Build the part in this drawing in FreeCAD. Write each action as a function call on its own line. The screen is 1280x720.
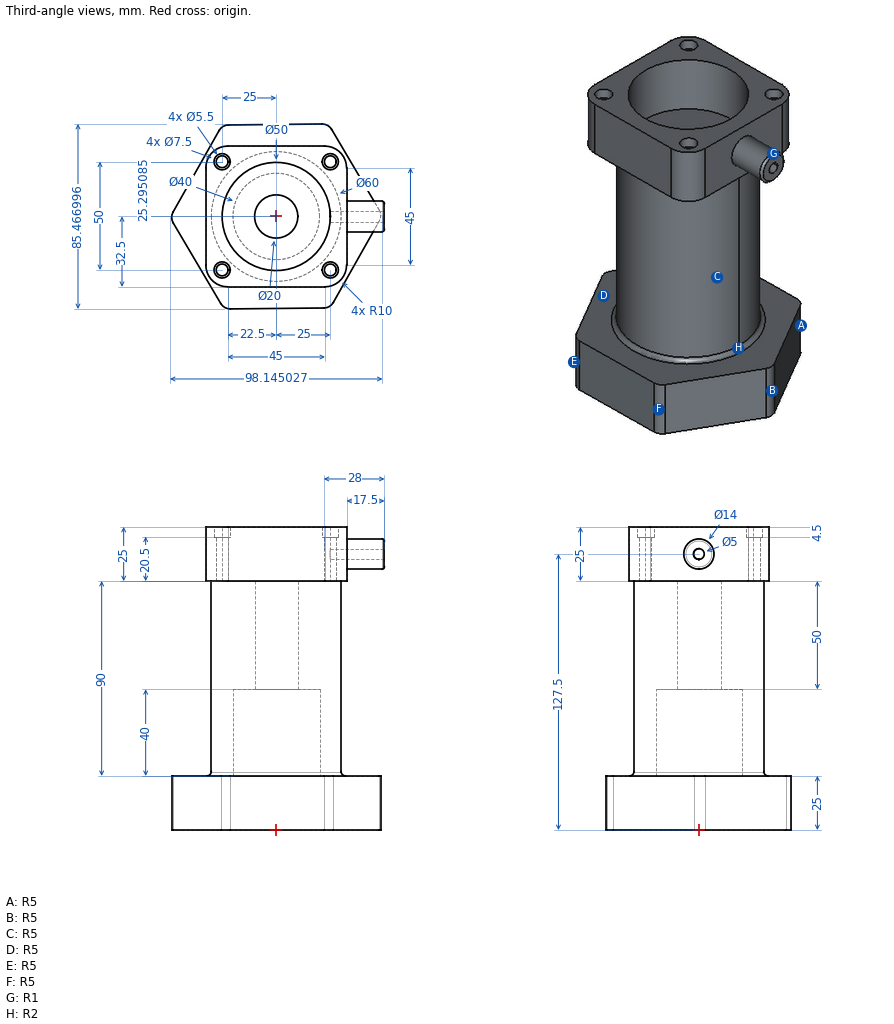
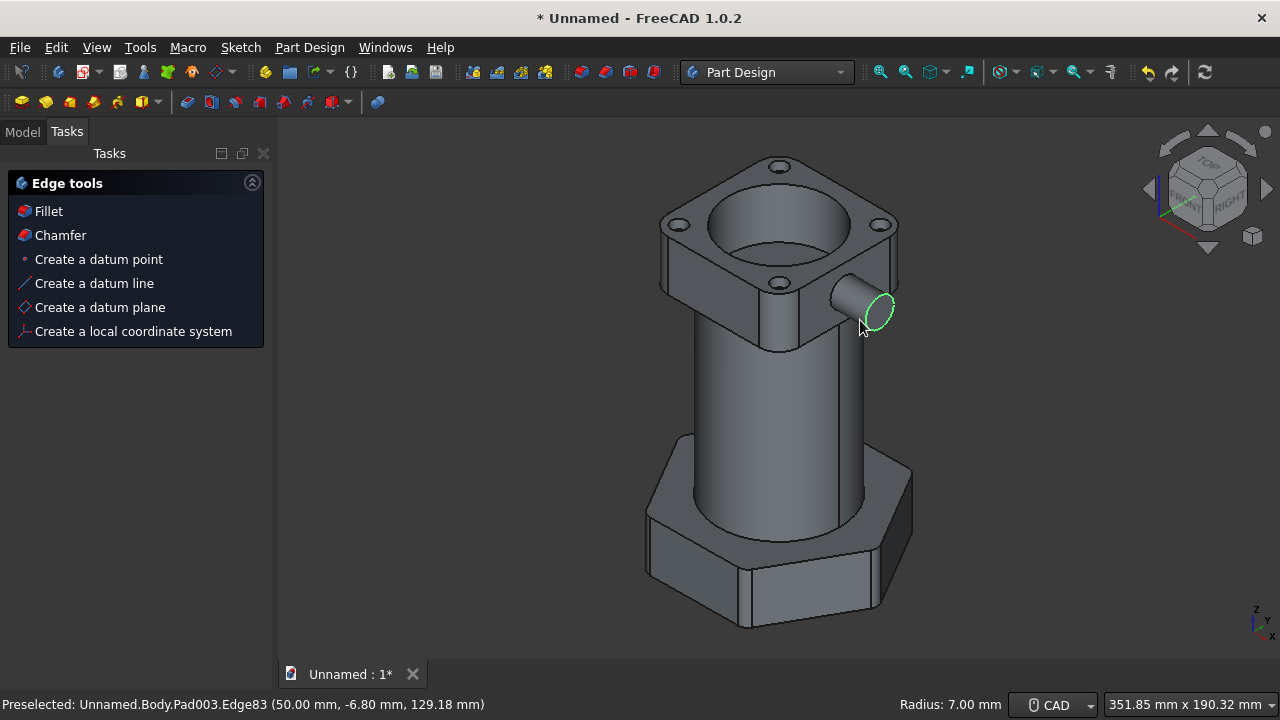
click(582, 72)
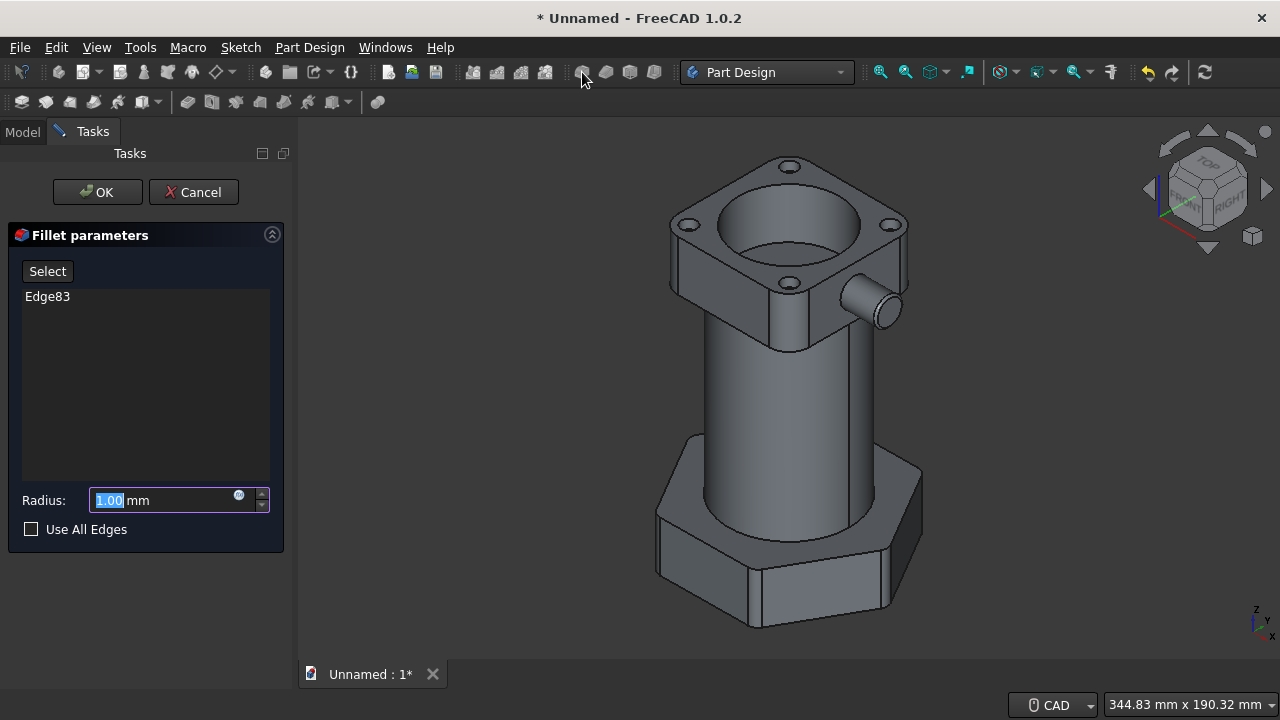
text(1)
key(Tab)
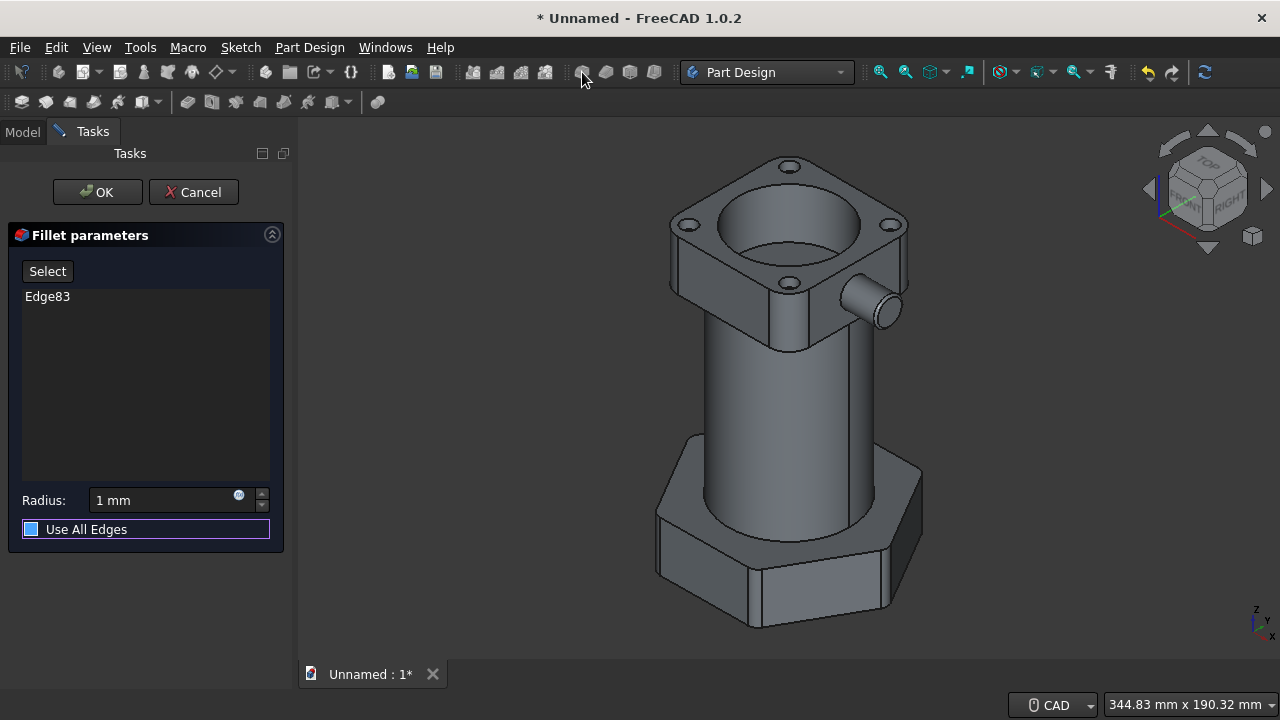
click(98, 192)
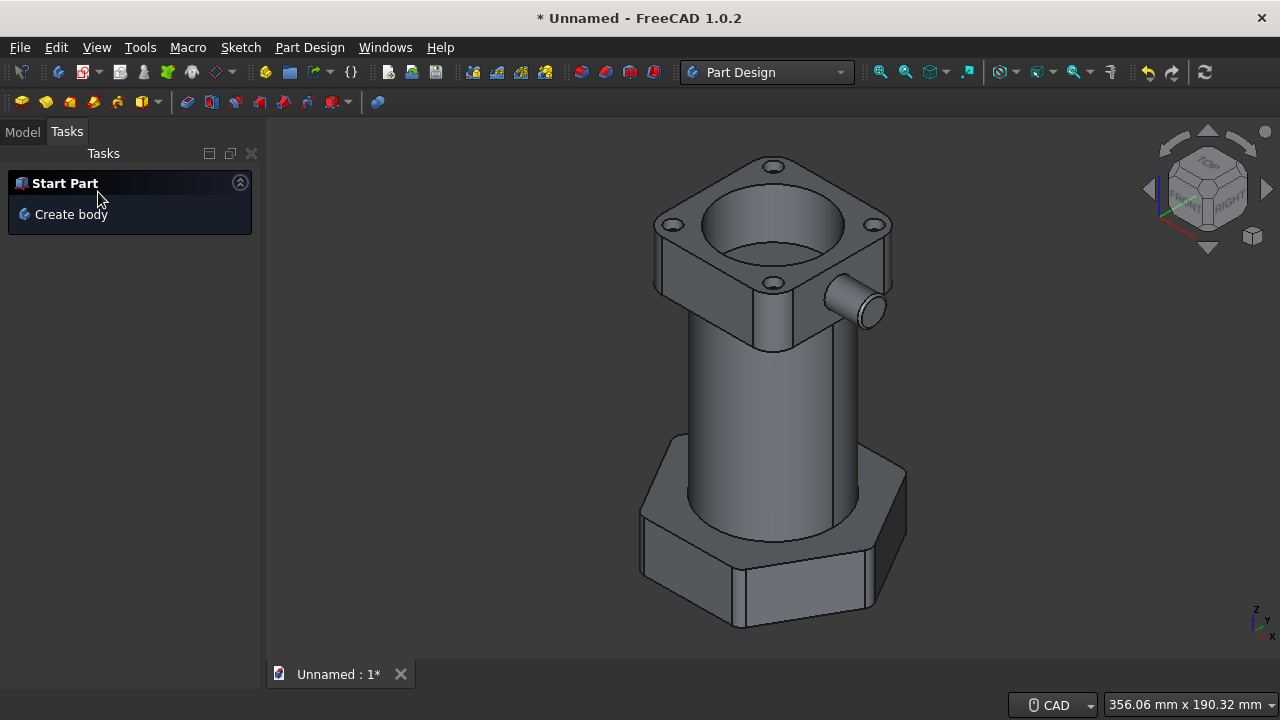
click(874, 311)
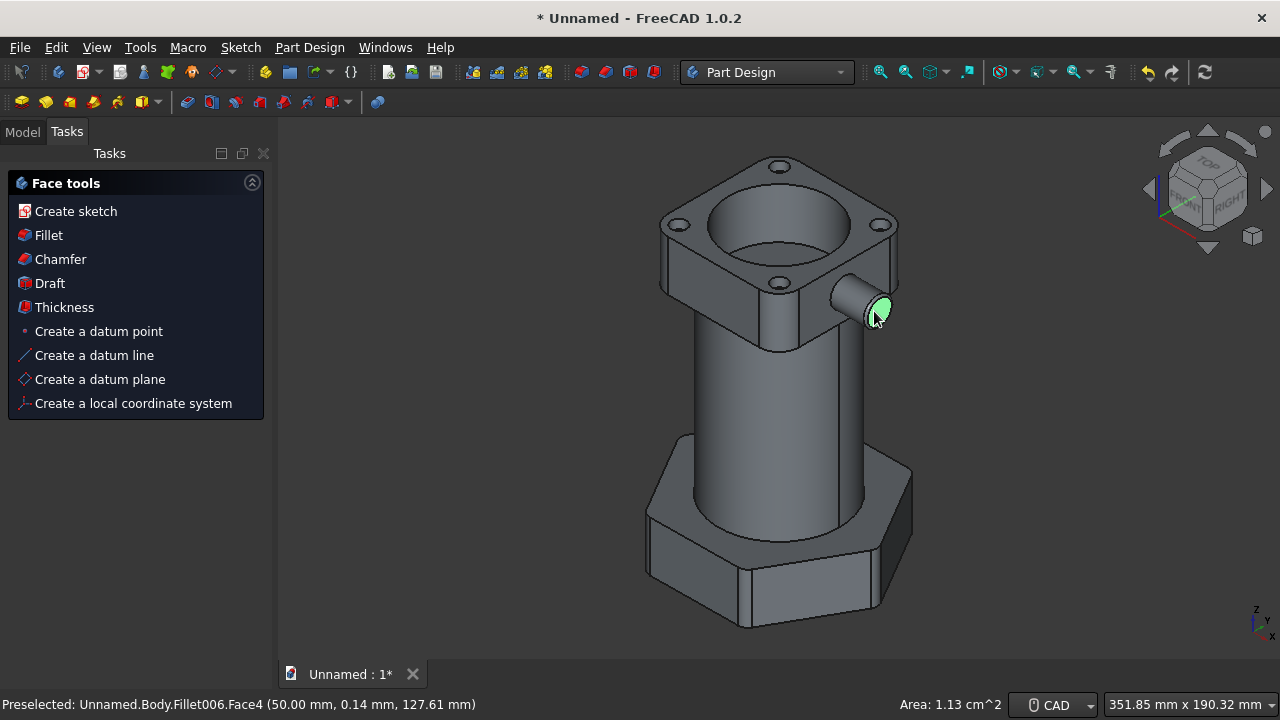
click(84, 72)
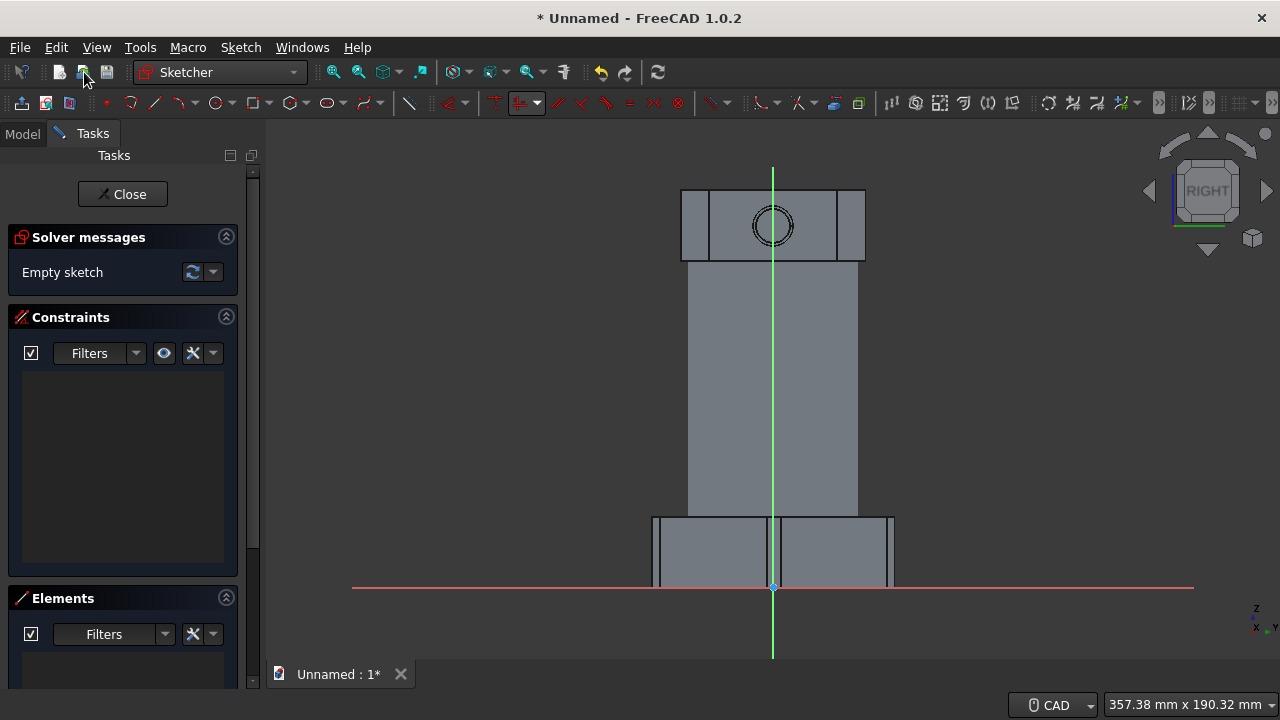
scroll(777, 217, up, 15)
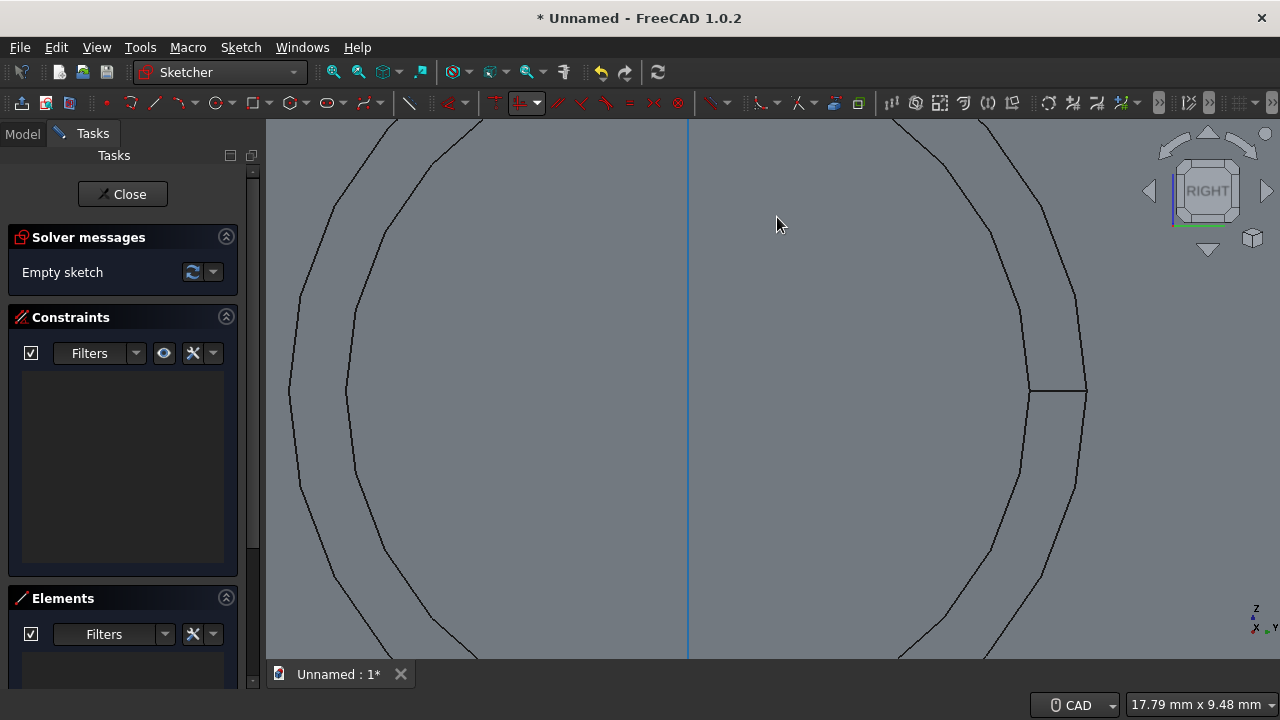
key(g)
key(c)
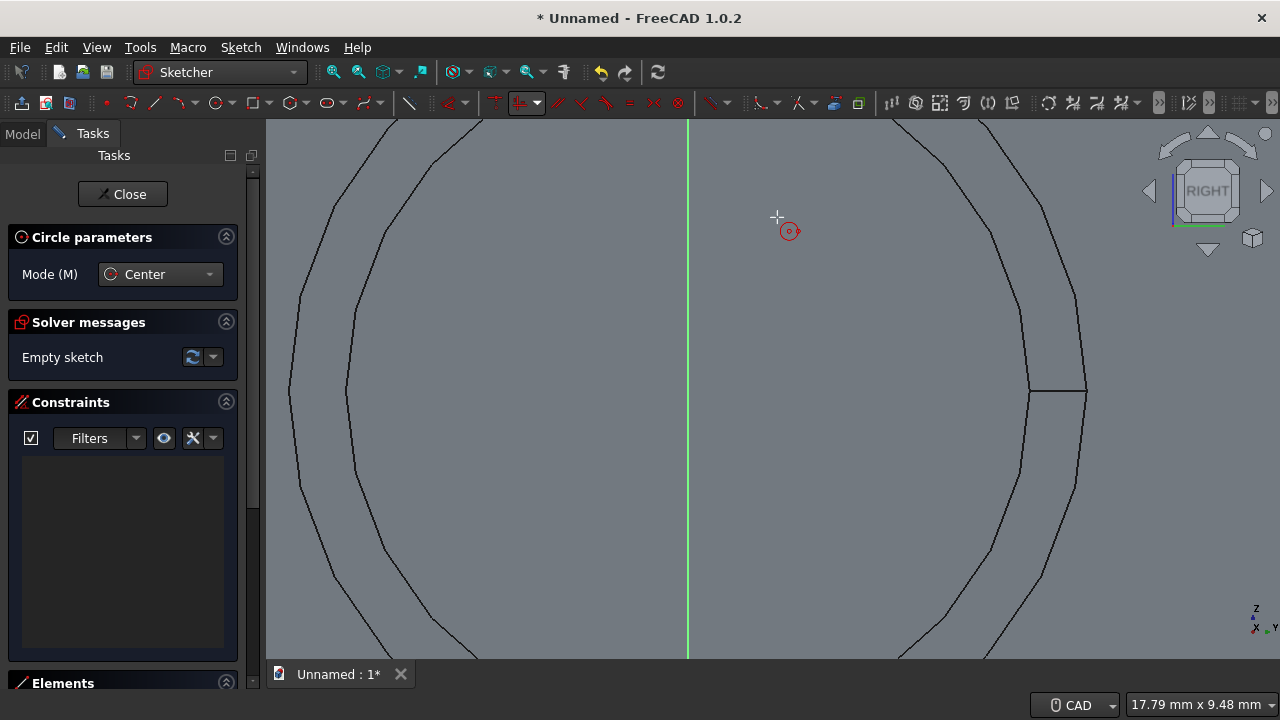
click(688, 391)
click(789, 291)
key(Escape)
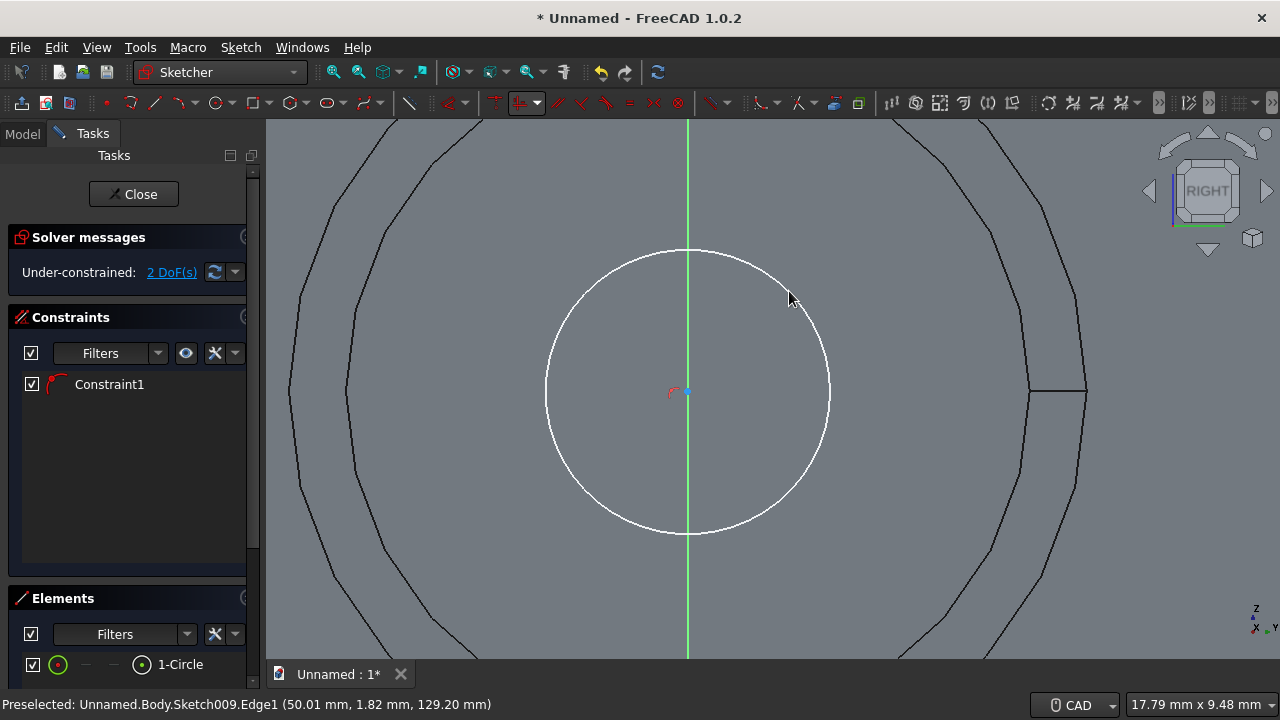
click(448, 104)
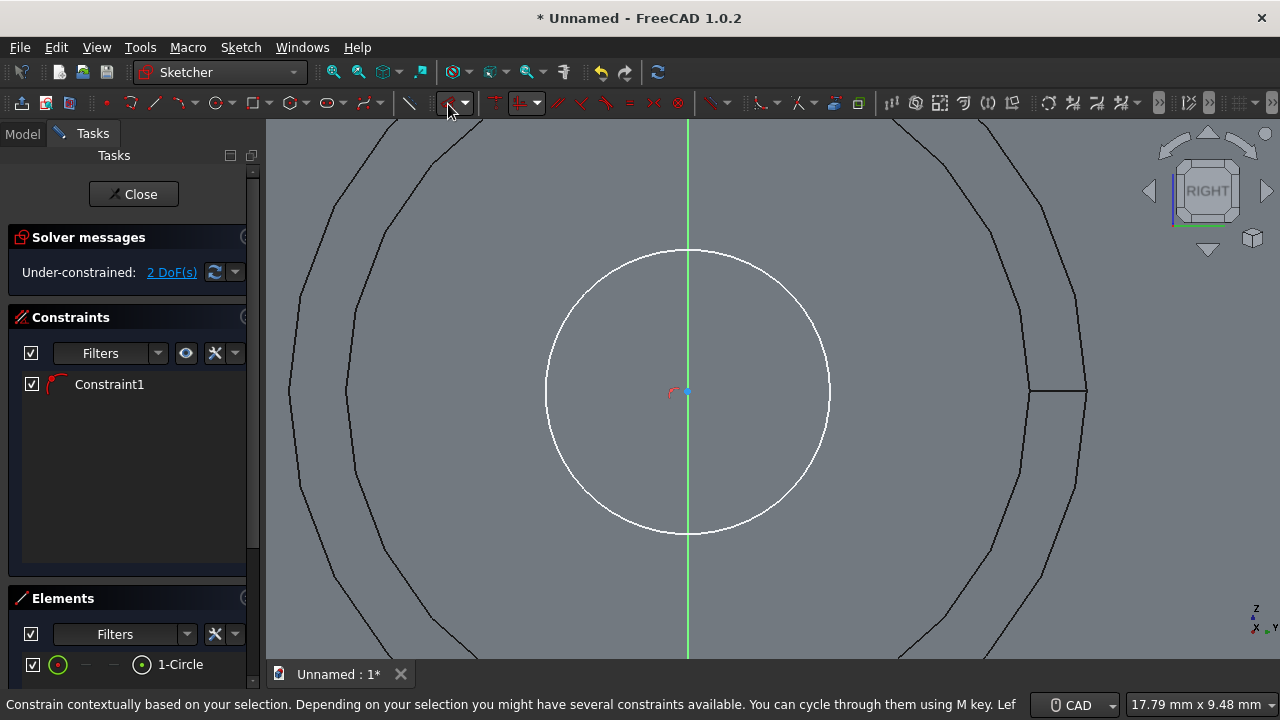
click(788, 291)
click(811, 268)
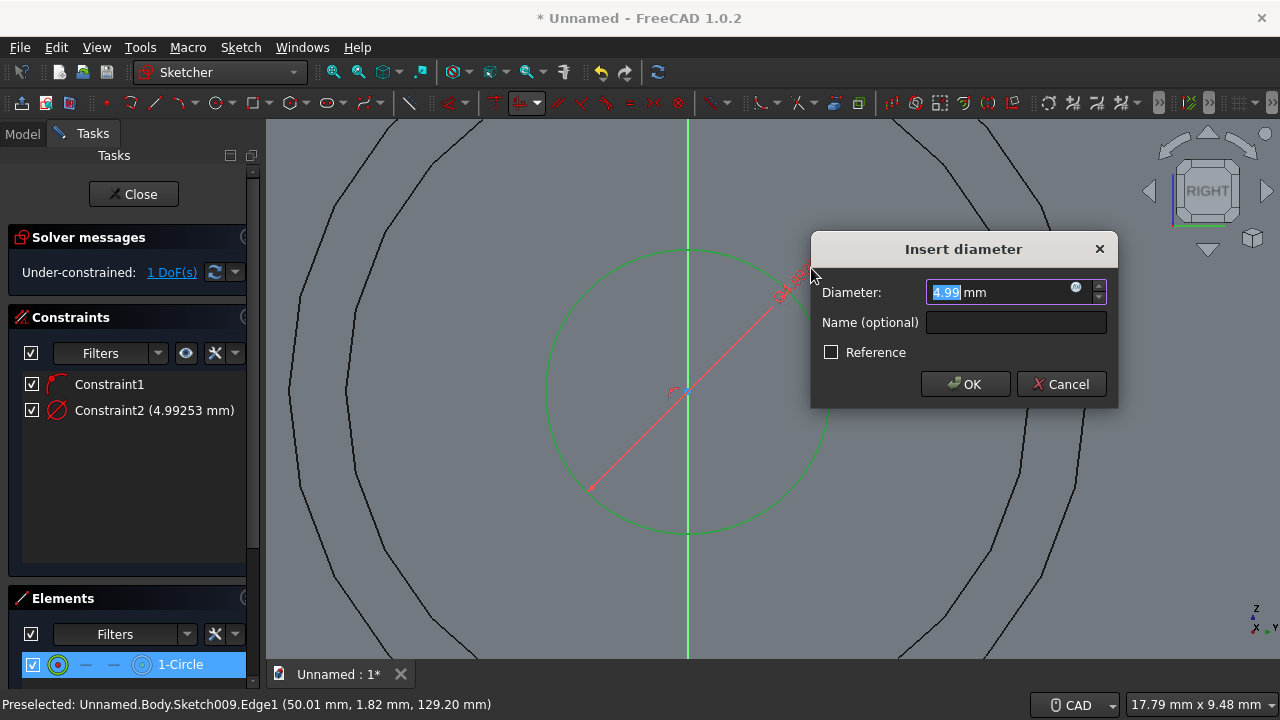
text(5)
key(Return)